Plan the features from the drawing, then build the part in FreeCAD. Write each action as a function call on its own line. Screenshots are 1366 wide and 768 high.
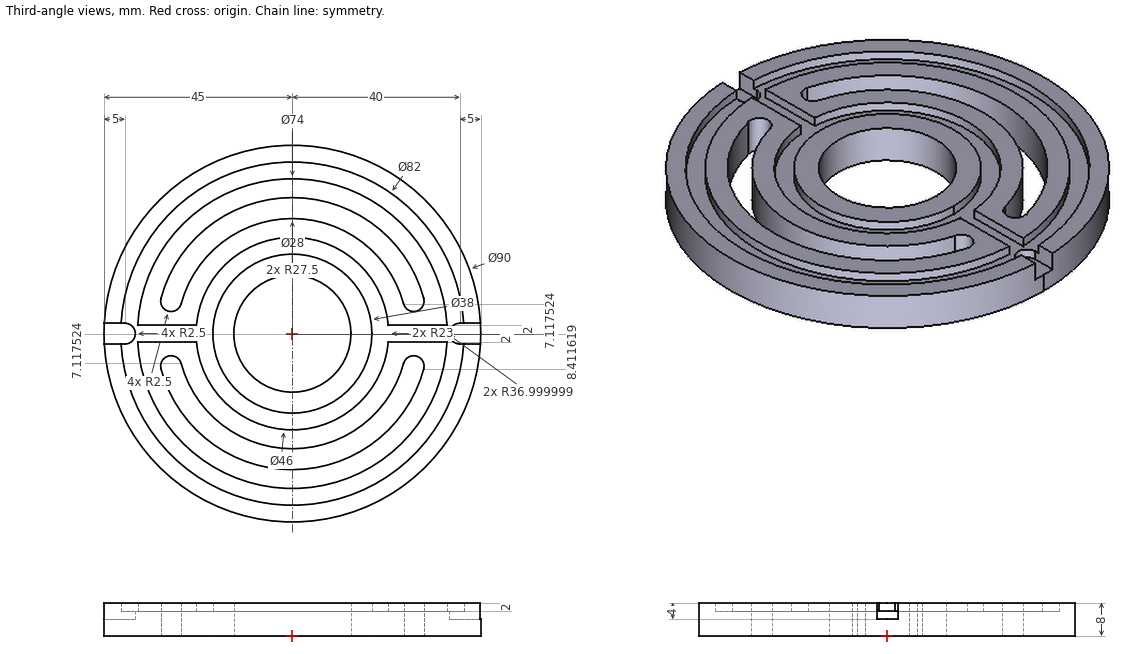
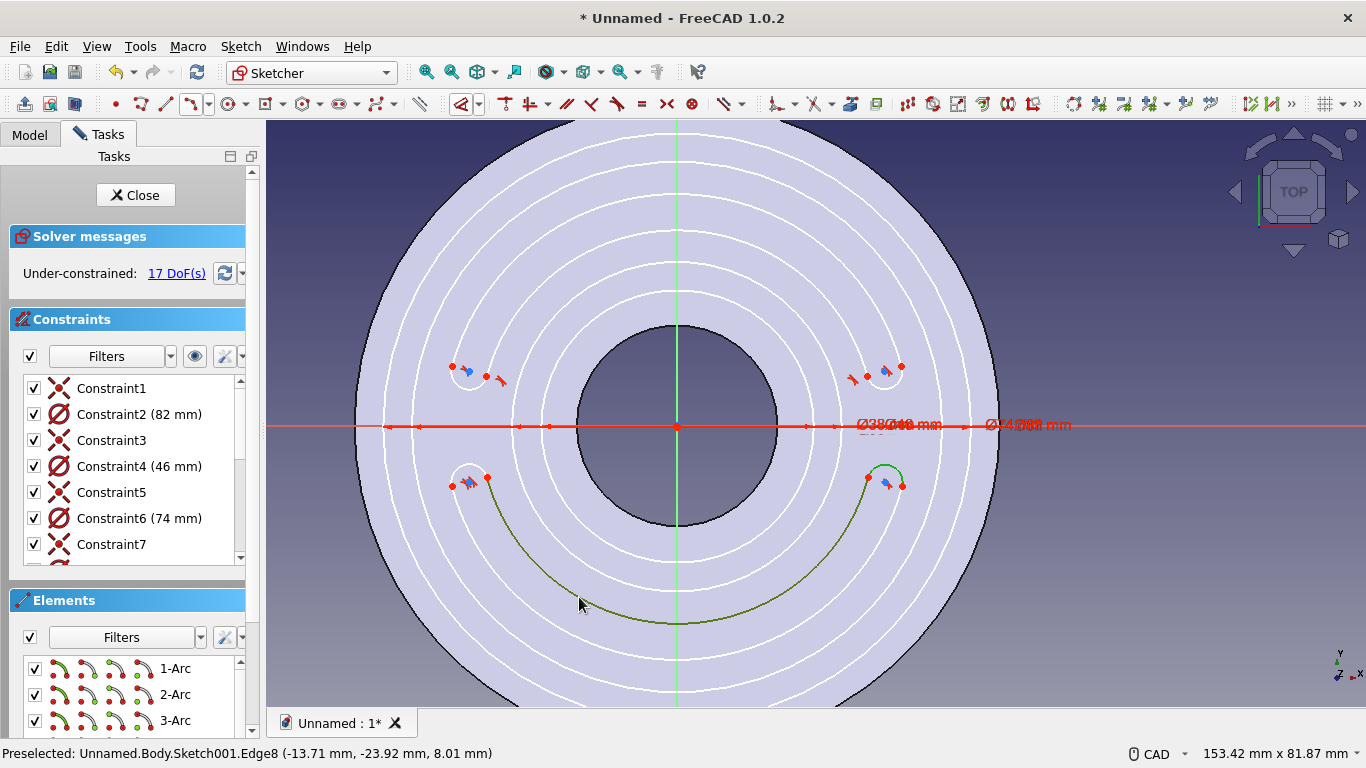
click(617, 104)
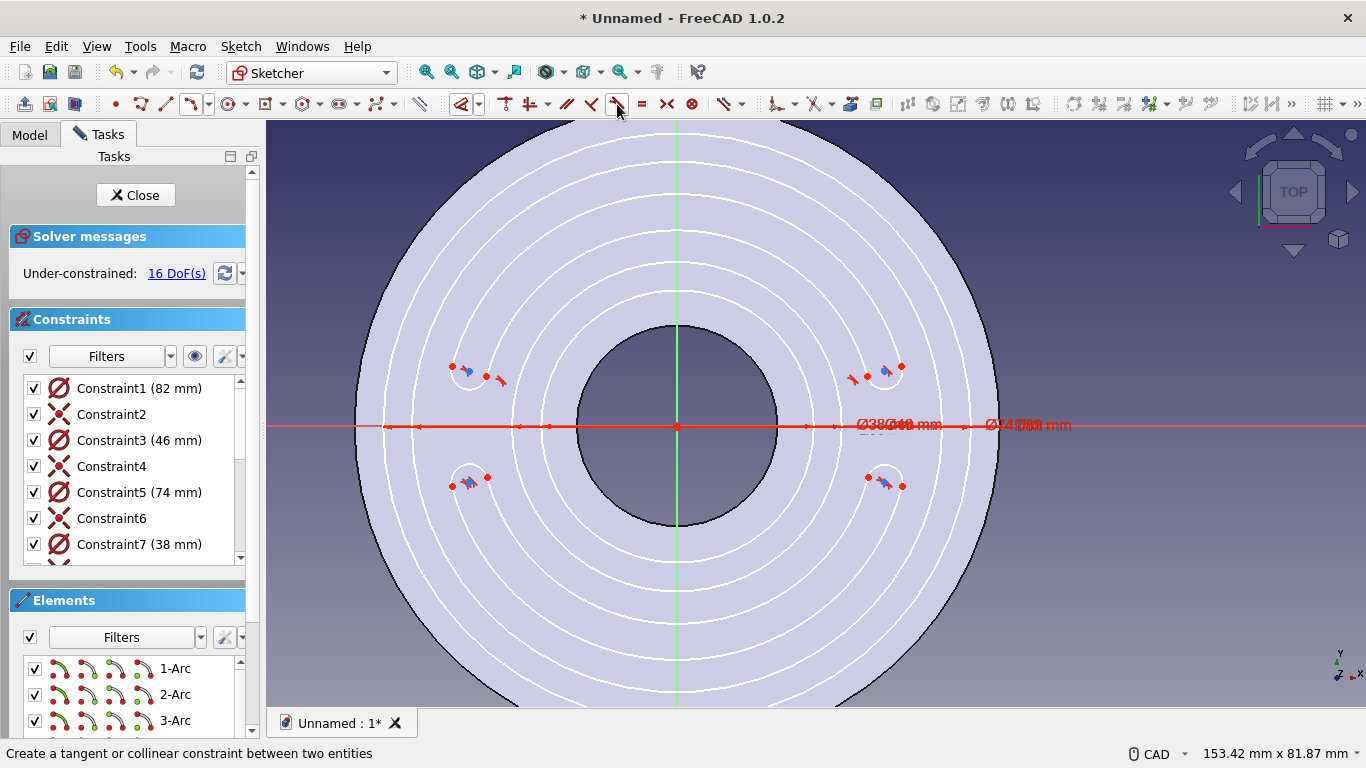
click(884, 219)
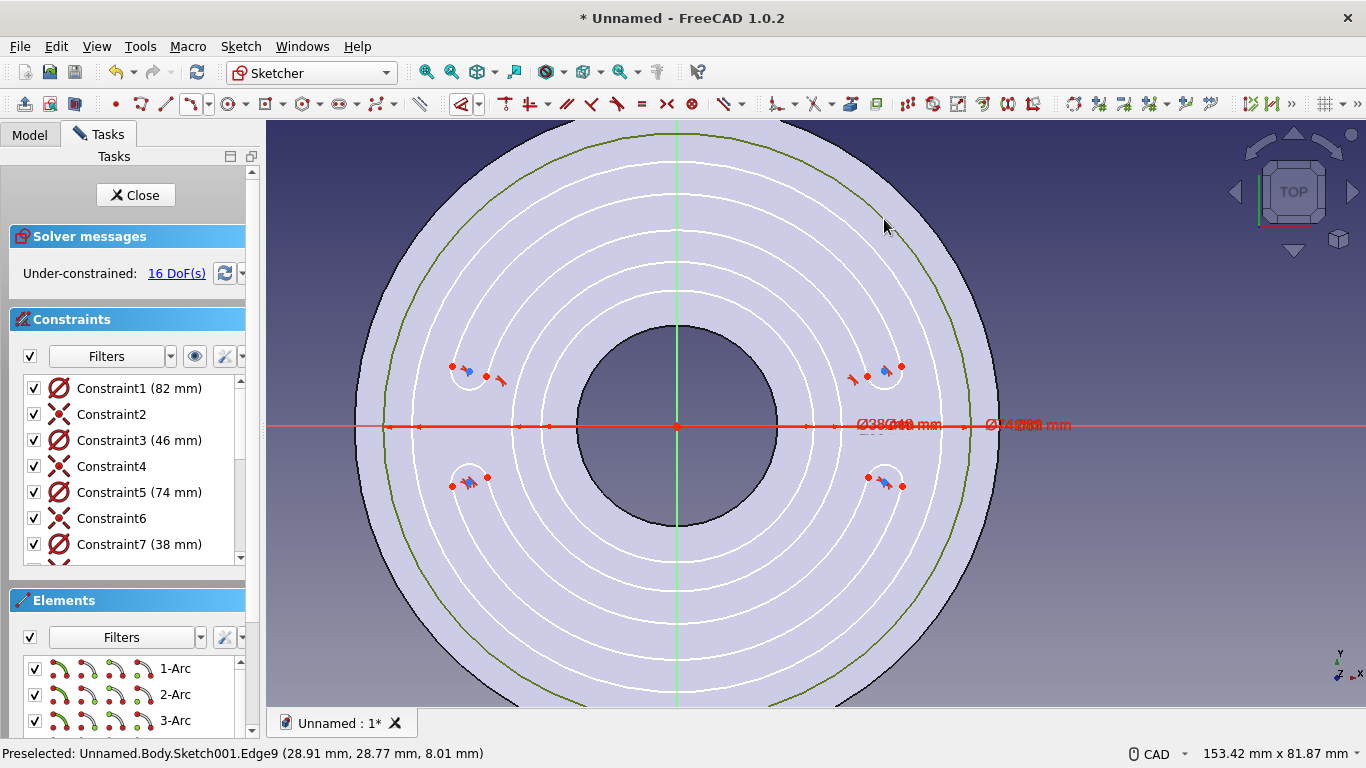
click(793, 225)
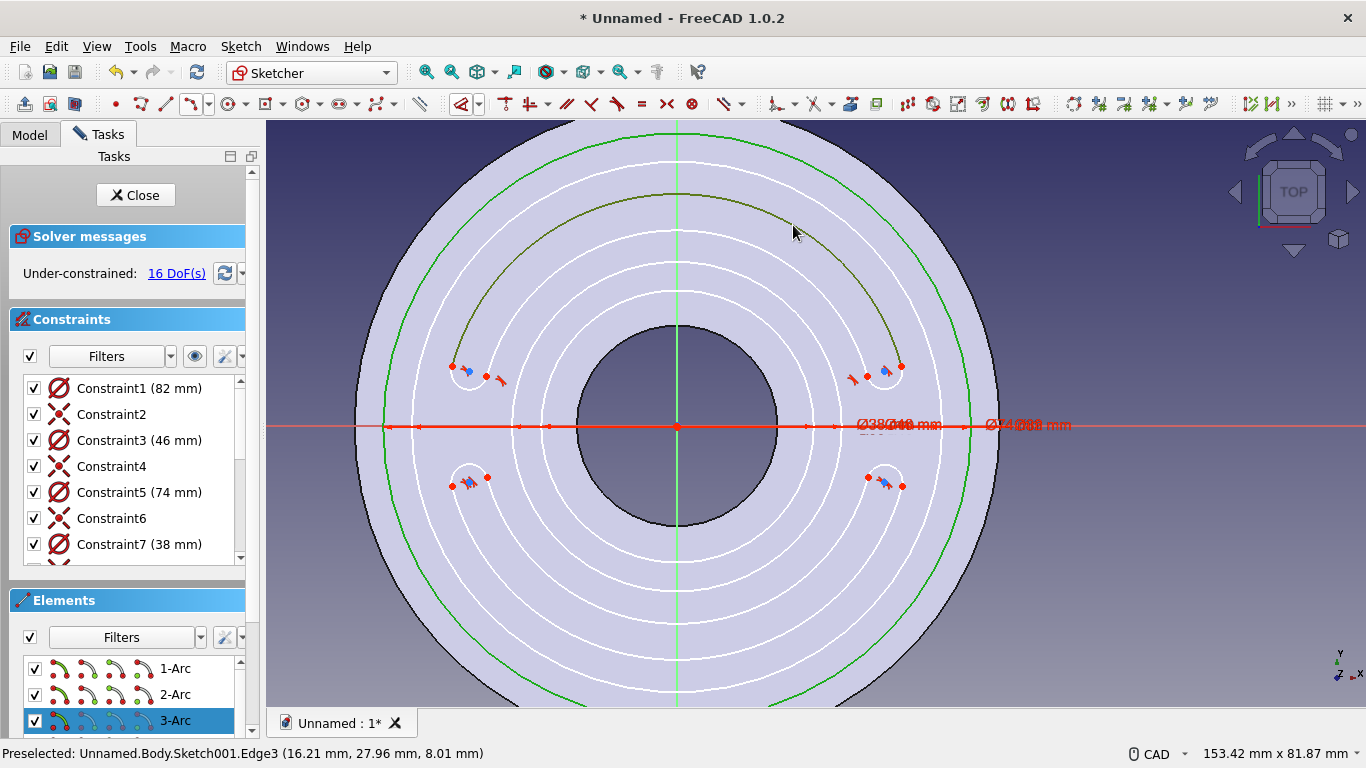
click(505, 104)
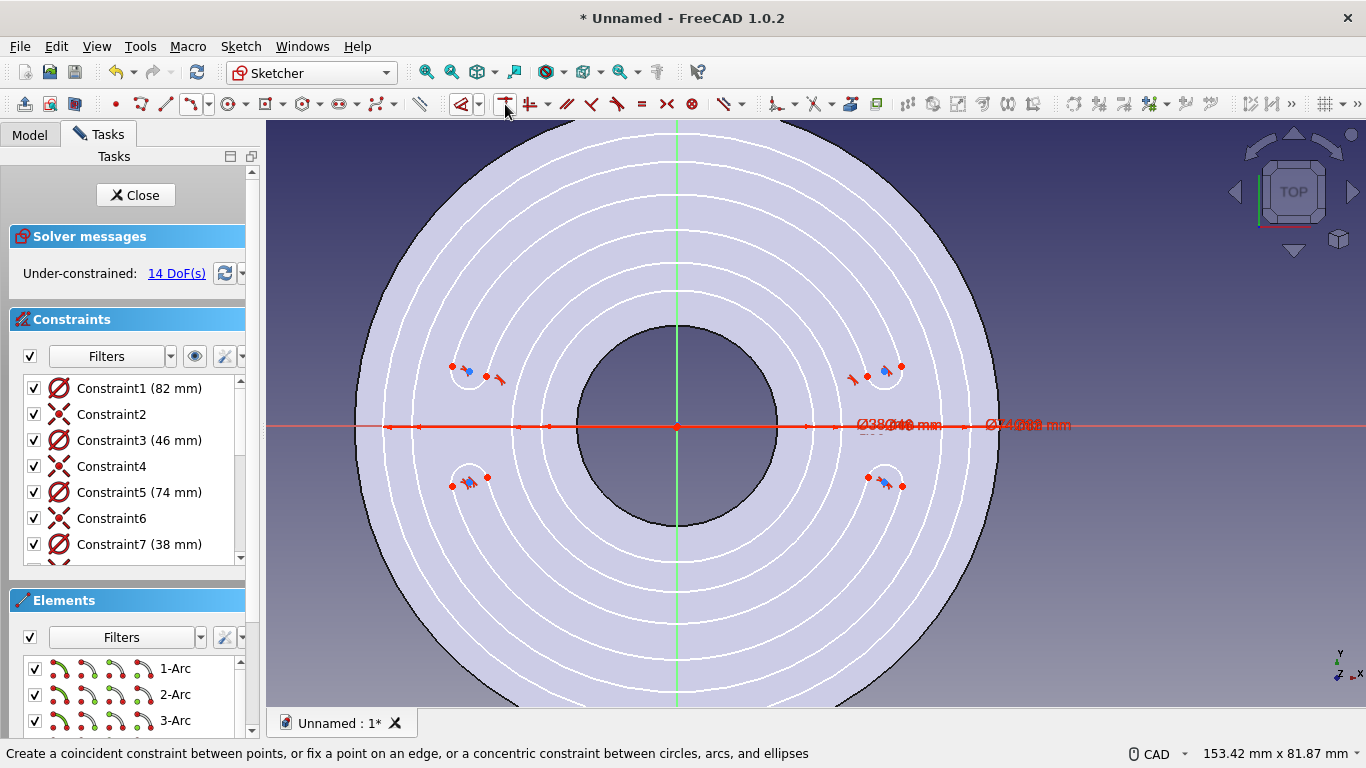
click(884, 219)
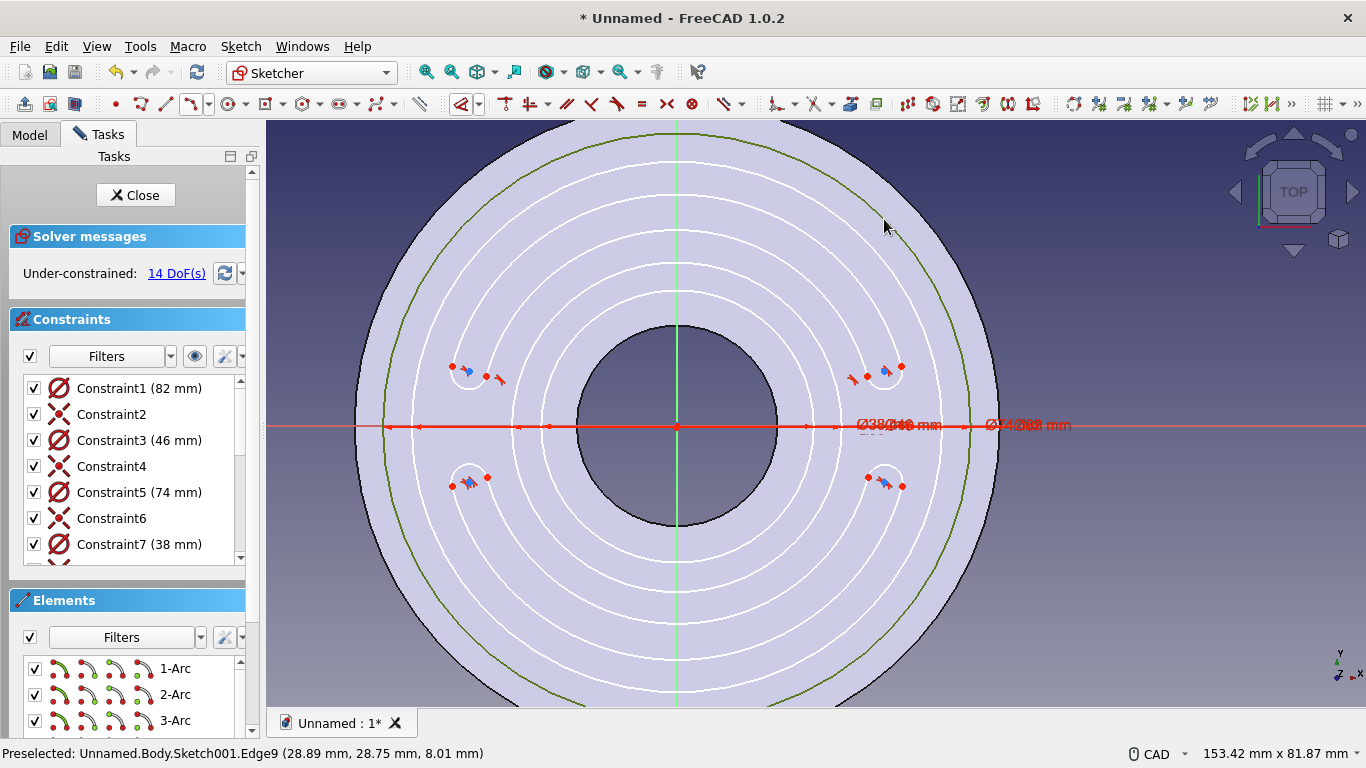
click(560, 629)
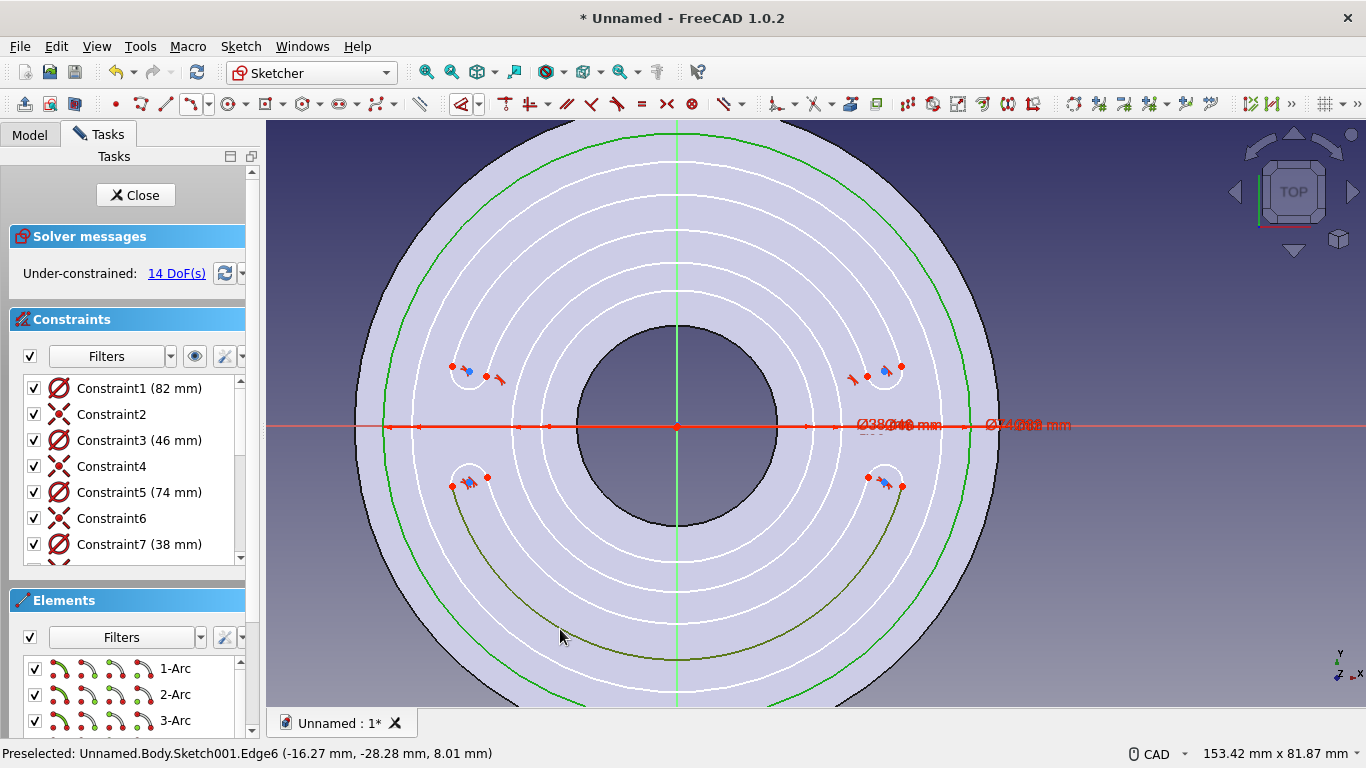
key(c)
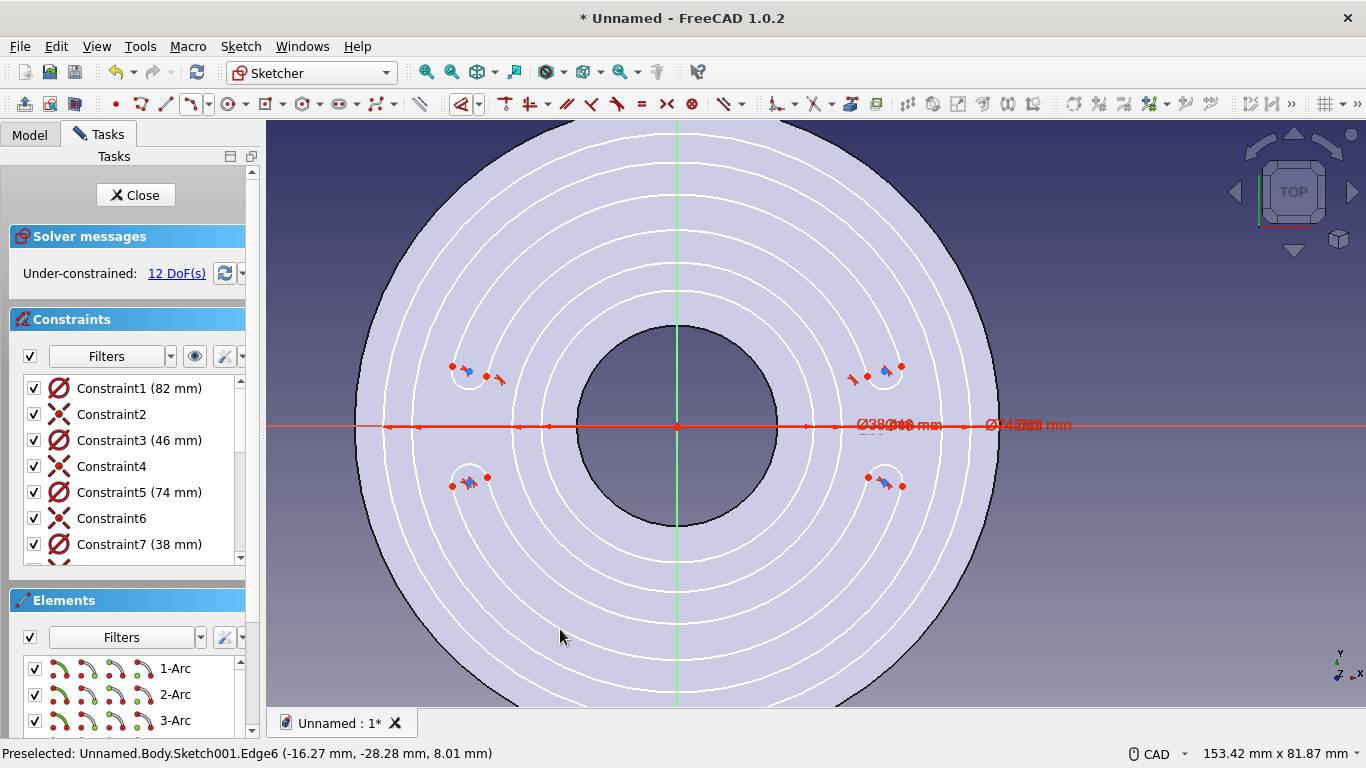
click(884, 219)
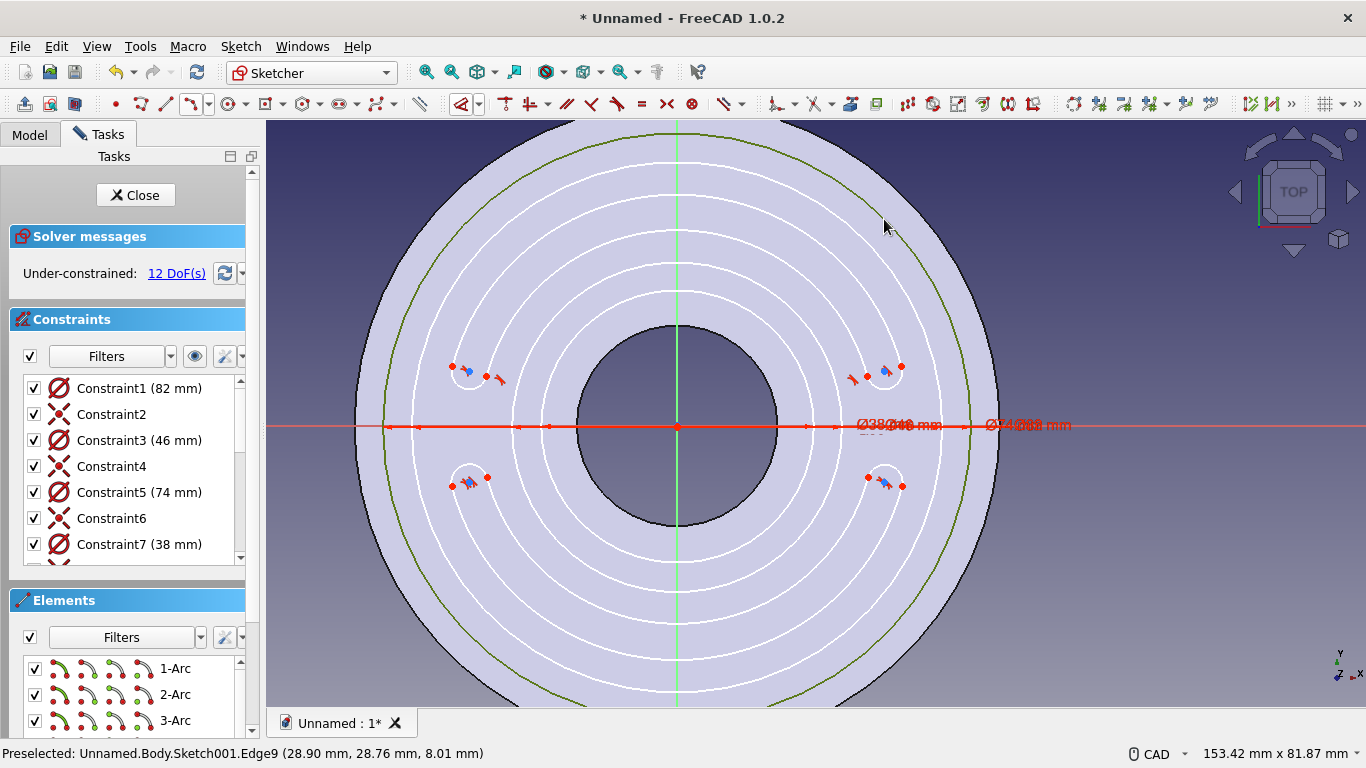
click(579, 597)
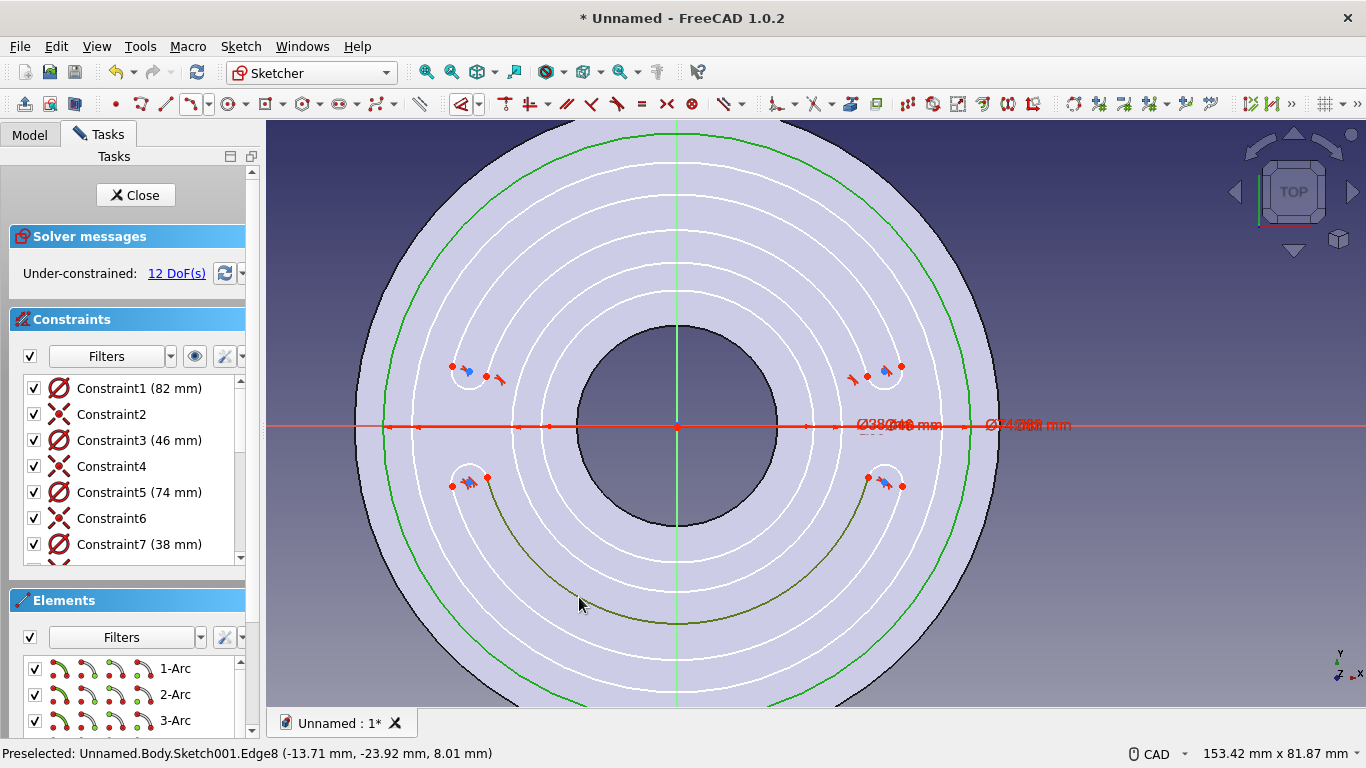
click(505, 104)